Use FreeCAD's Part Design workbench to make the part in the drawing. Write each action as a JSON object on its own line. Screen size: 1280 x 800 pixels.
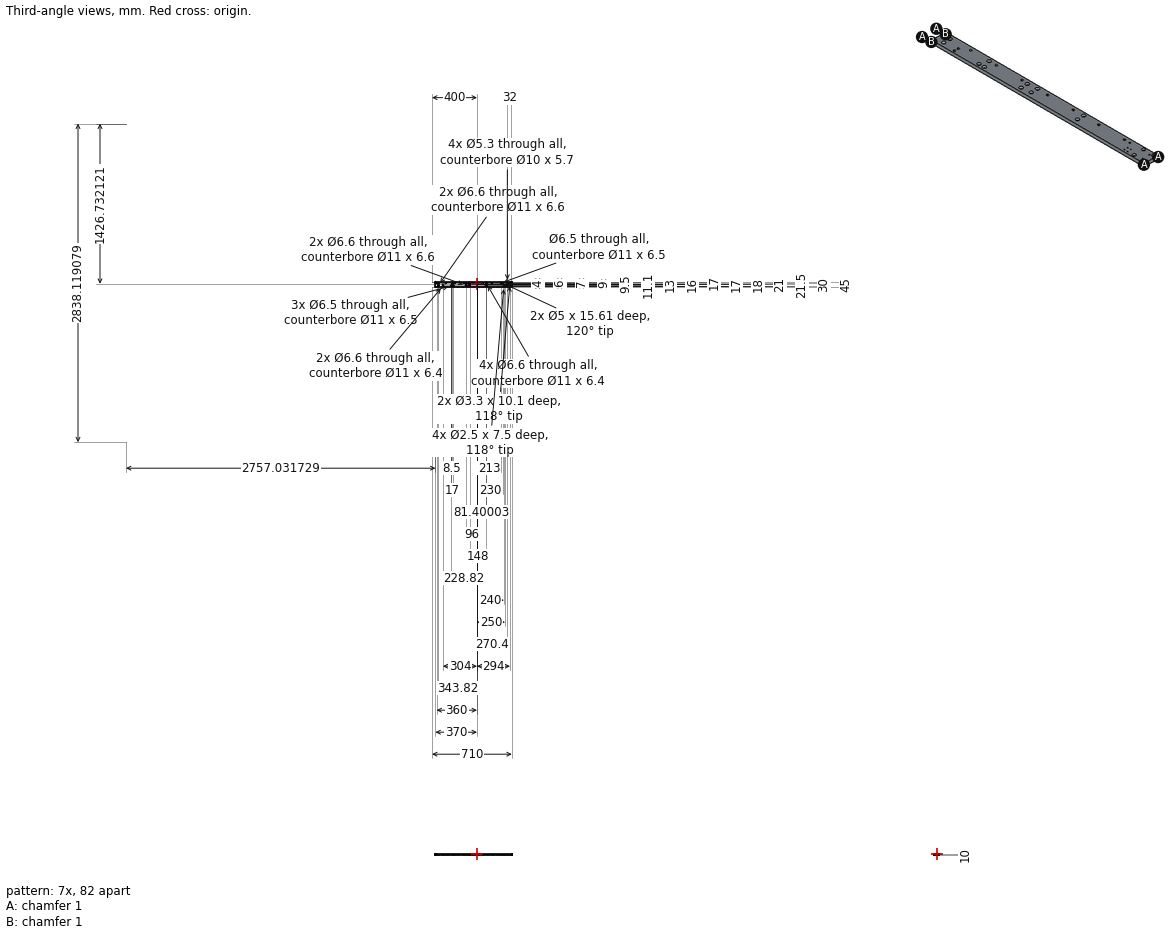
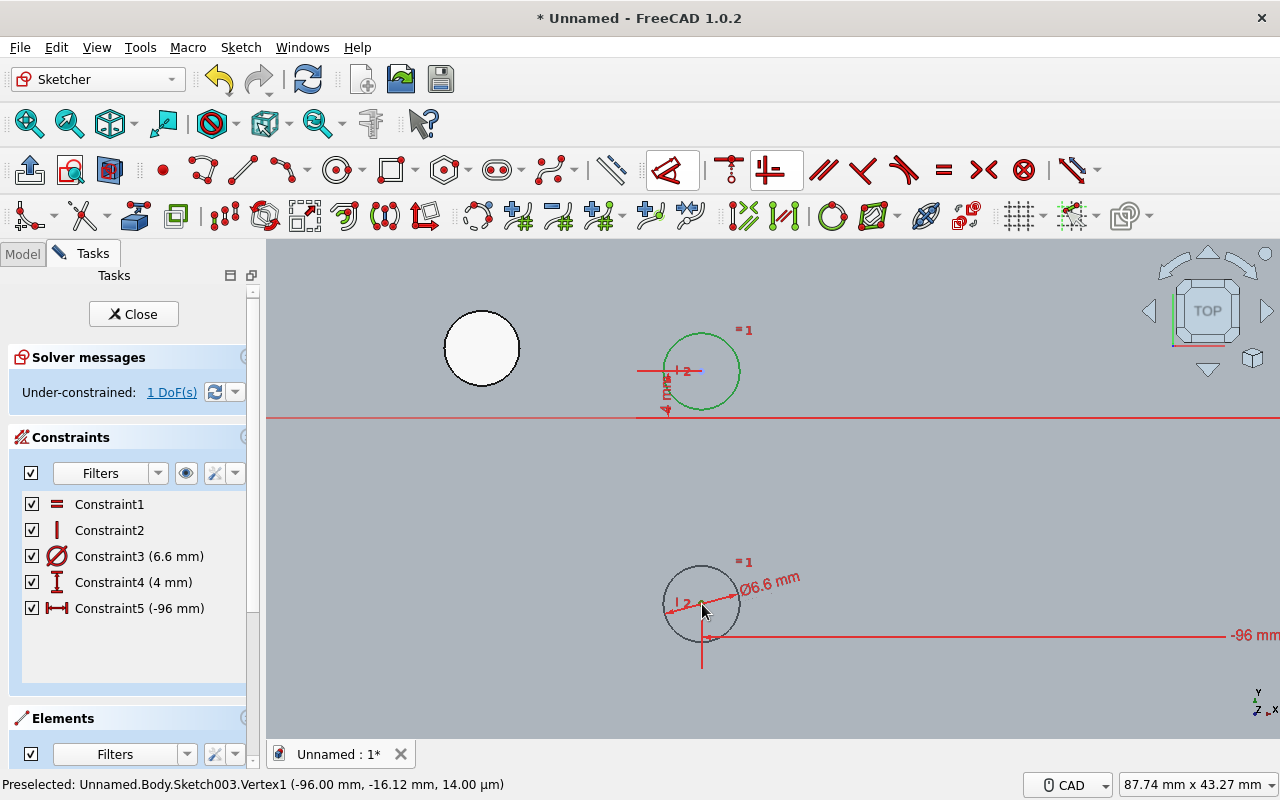
{"action": "left_click", "coordinate": [694, 170]}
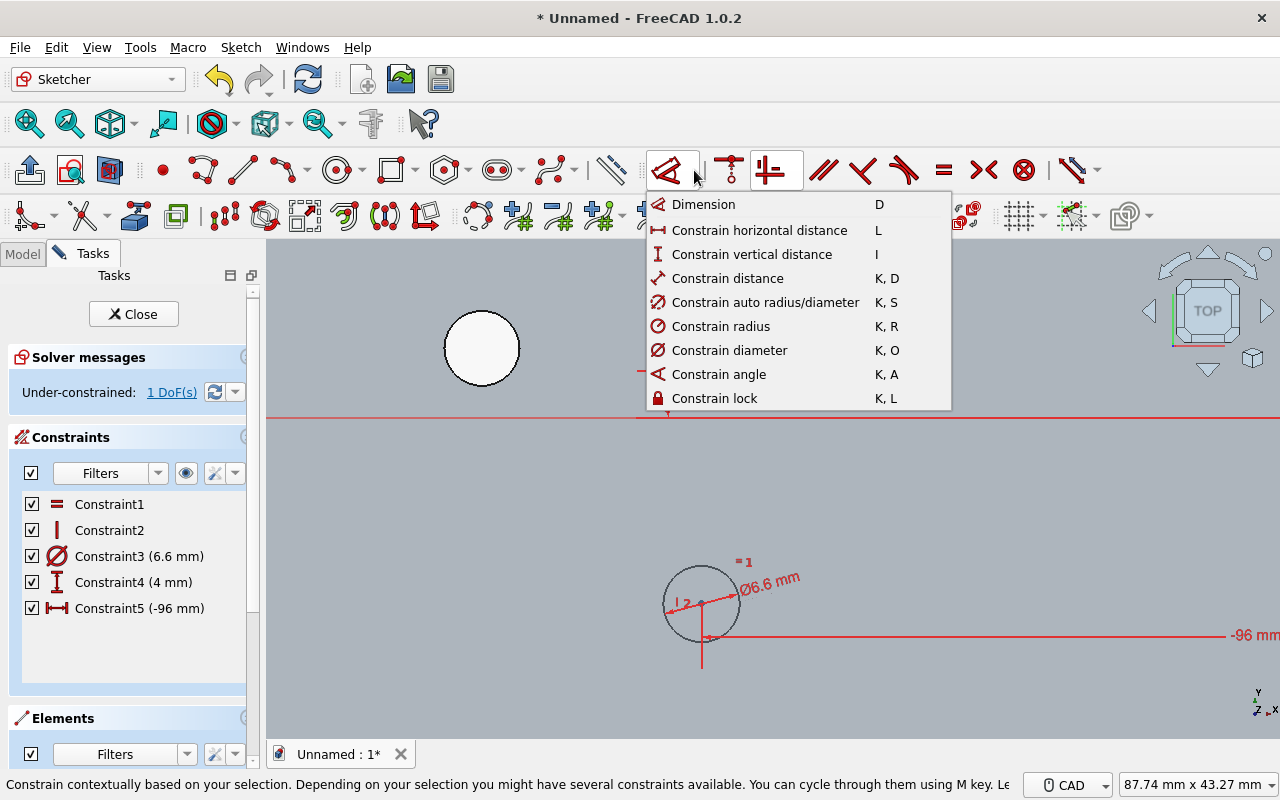
{"action": "left_click", "coordinate": [799, 254]}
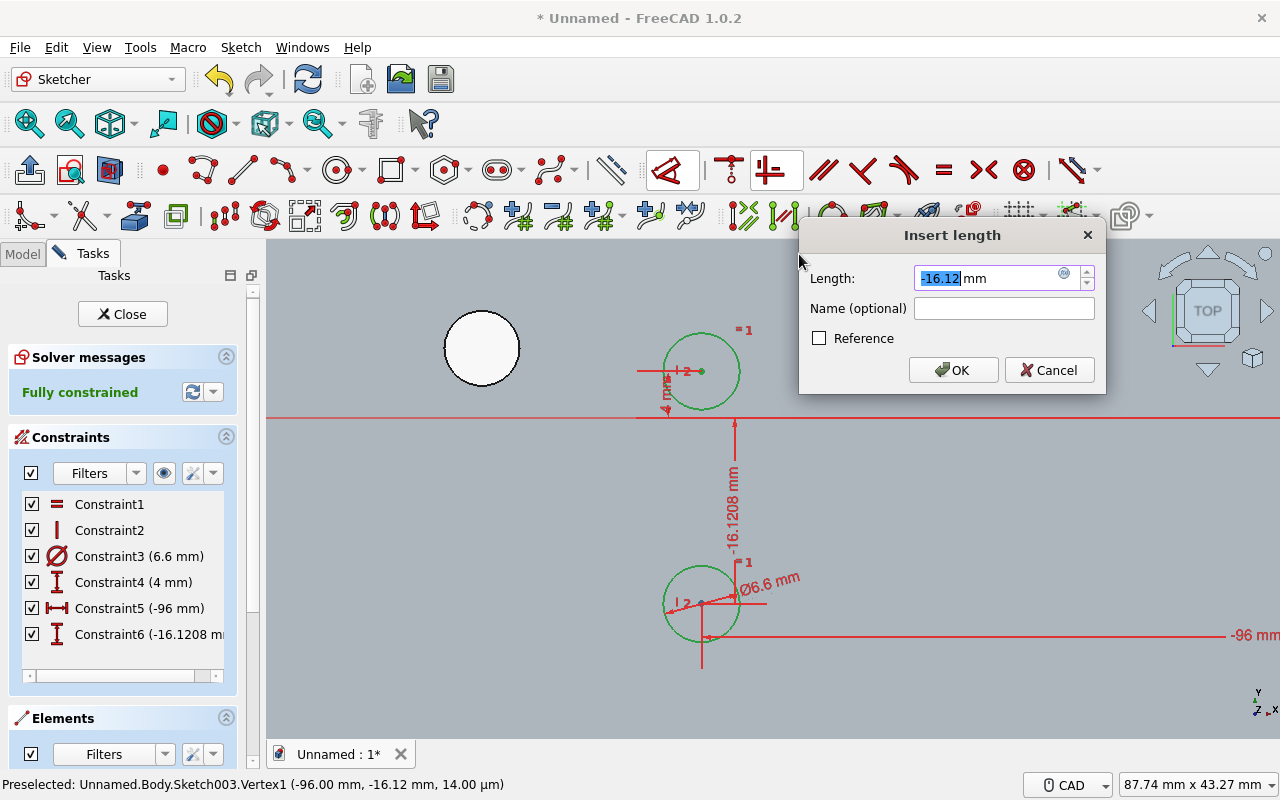
{"action": "type", "text": "-16"}
{"action": "key", "text": "Return"}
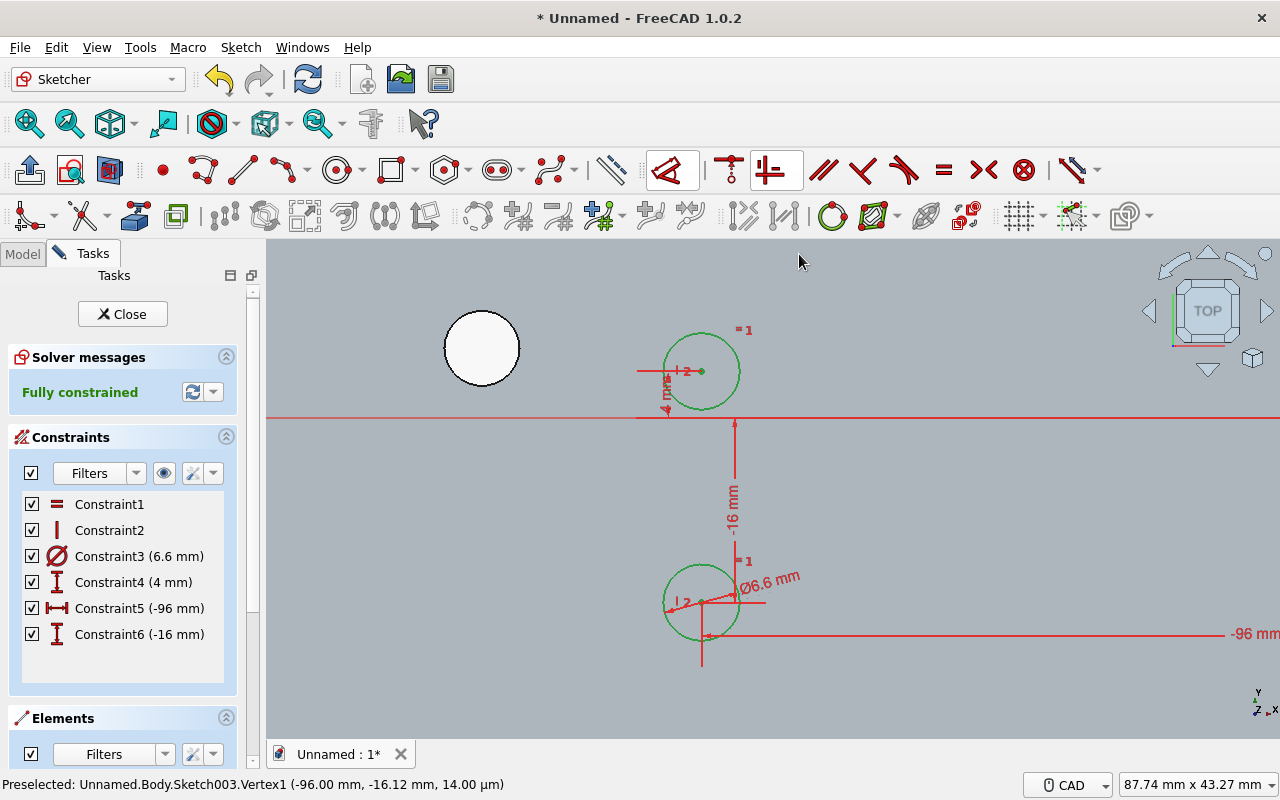
{"action": "left_click", "coordinate": [123, 314]}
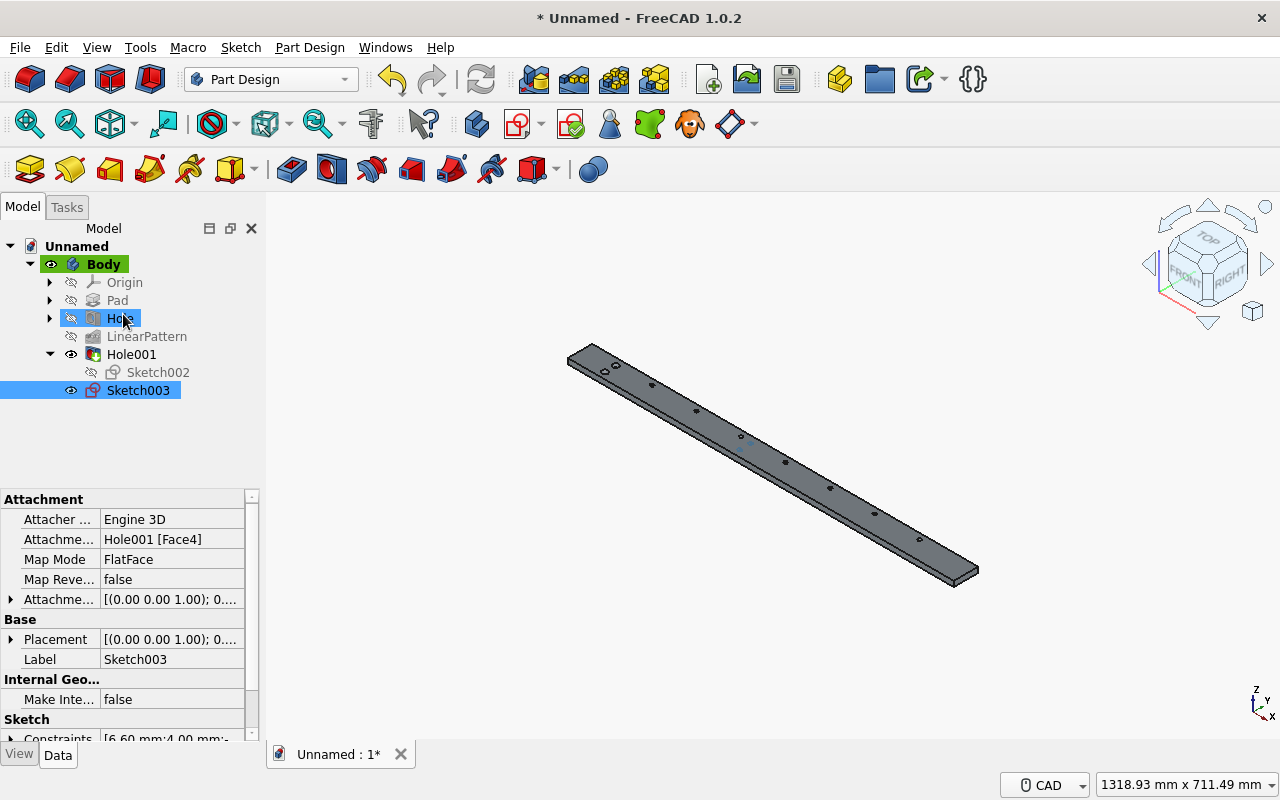
{"action": "left_click", "coordinate": [332, 170]}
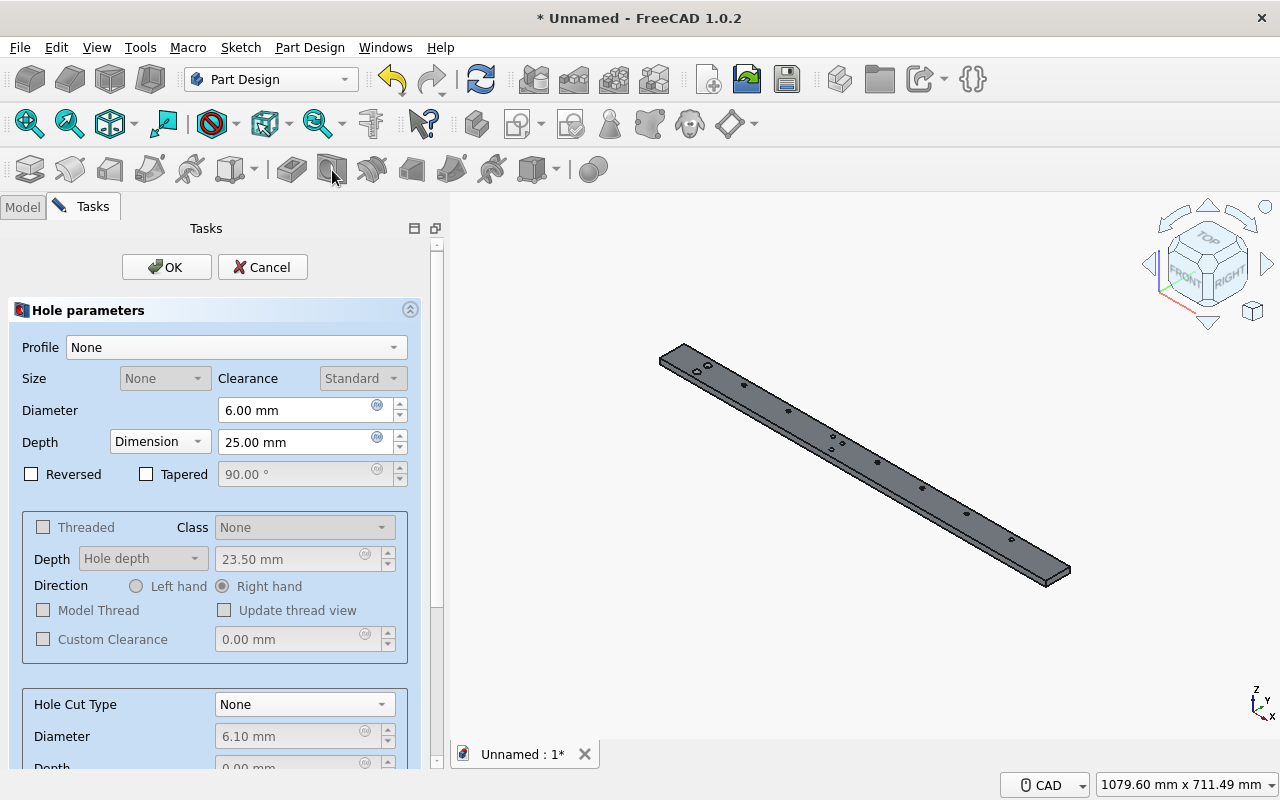
{"action": "triple_click", "coordinate": [305, 410]}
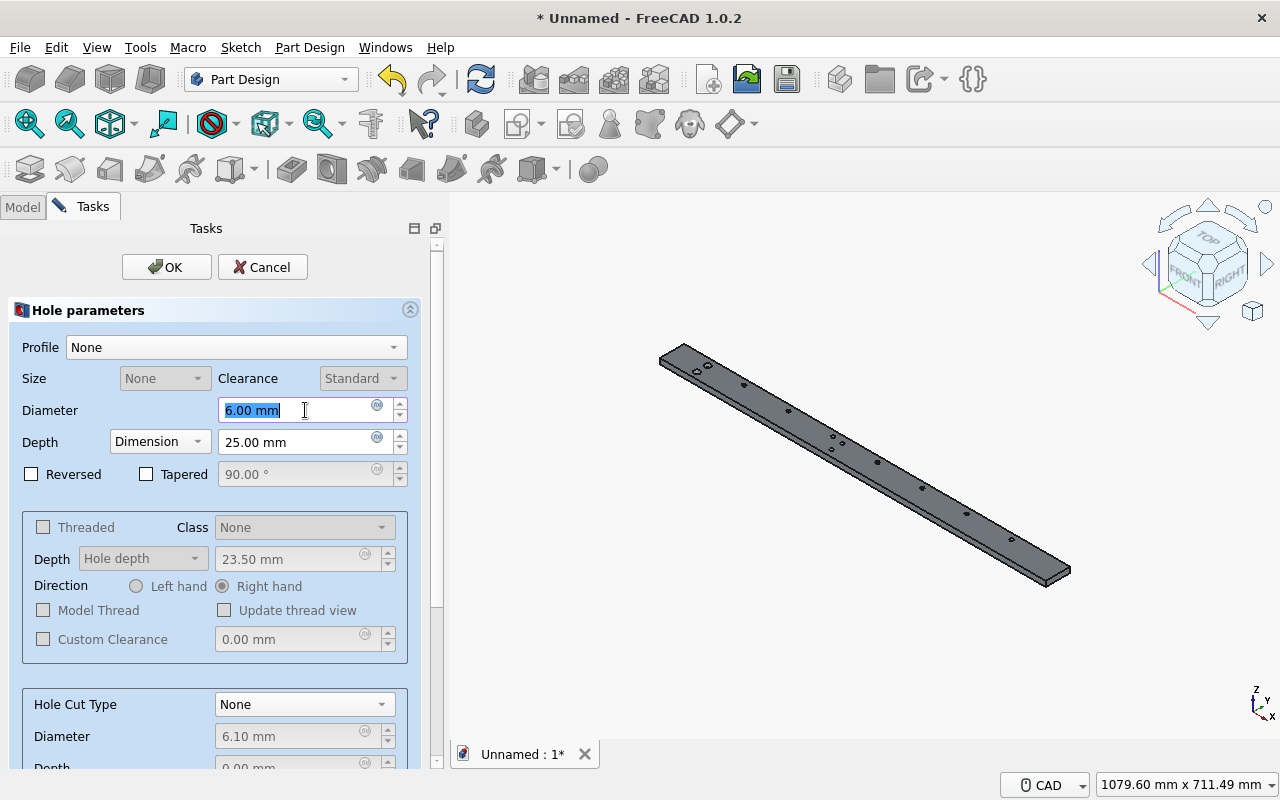
{"action": "type", "text": "6.6"}
{"action": "key", "text": "Tab"}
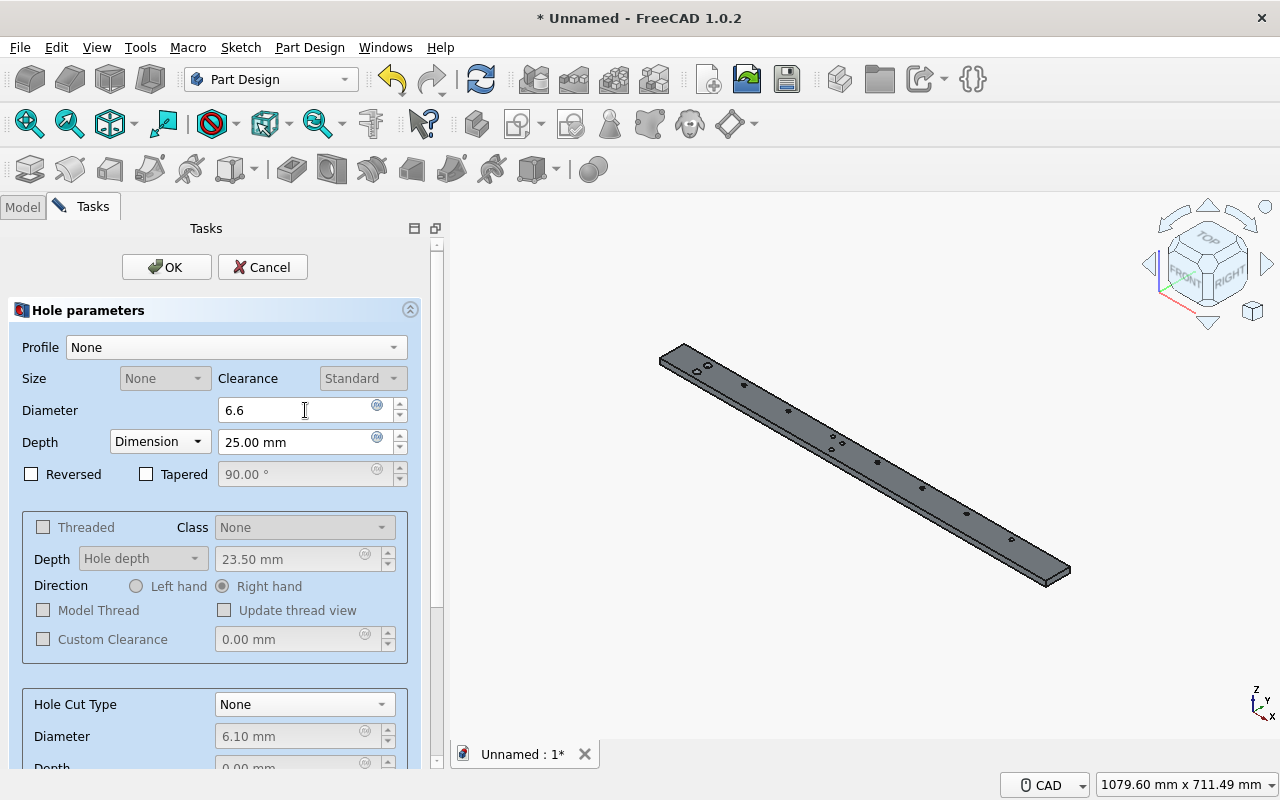
{"action": "left_click", "coordinate": [161, 442]}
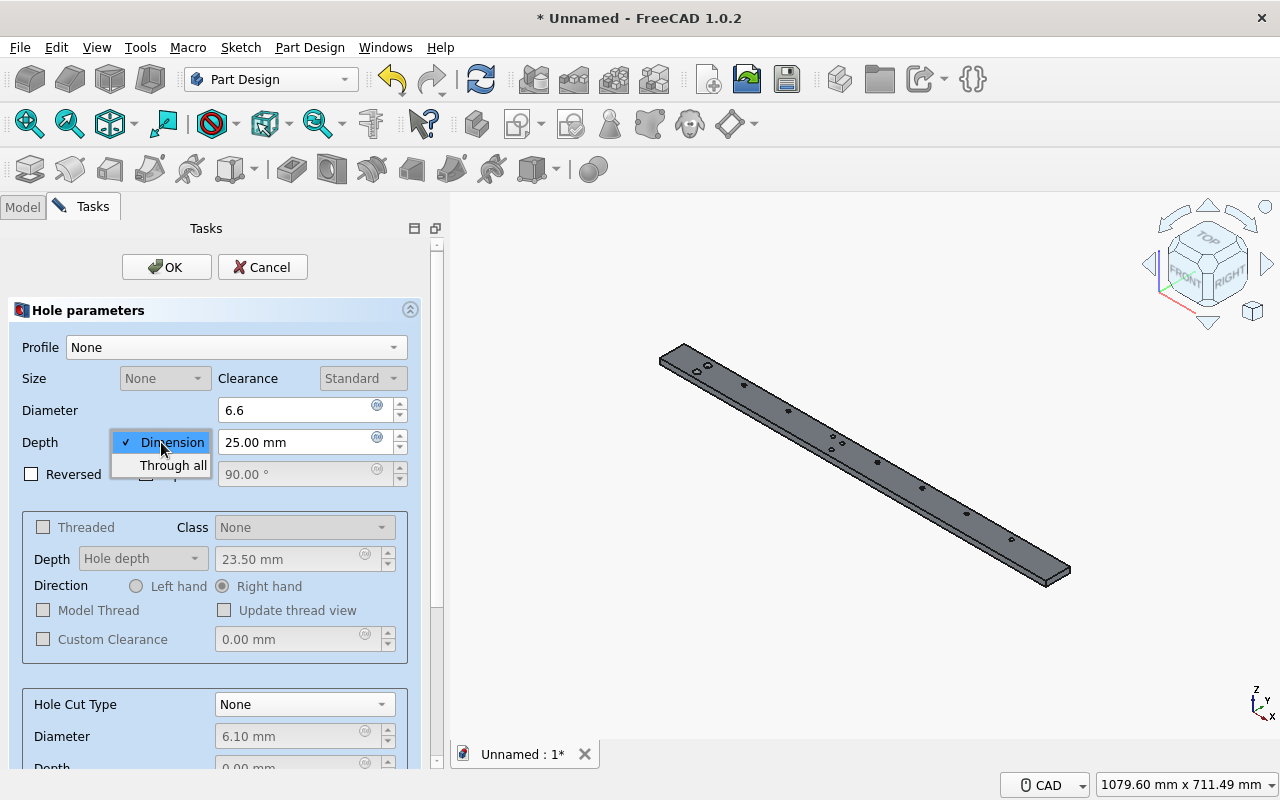
{"action": "left_click", "coordinate": [160, 466]}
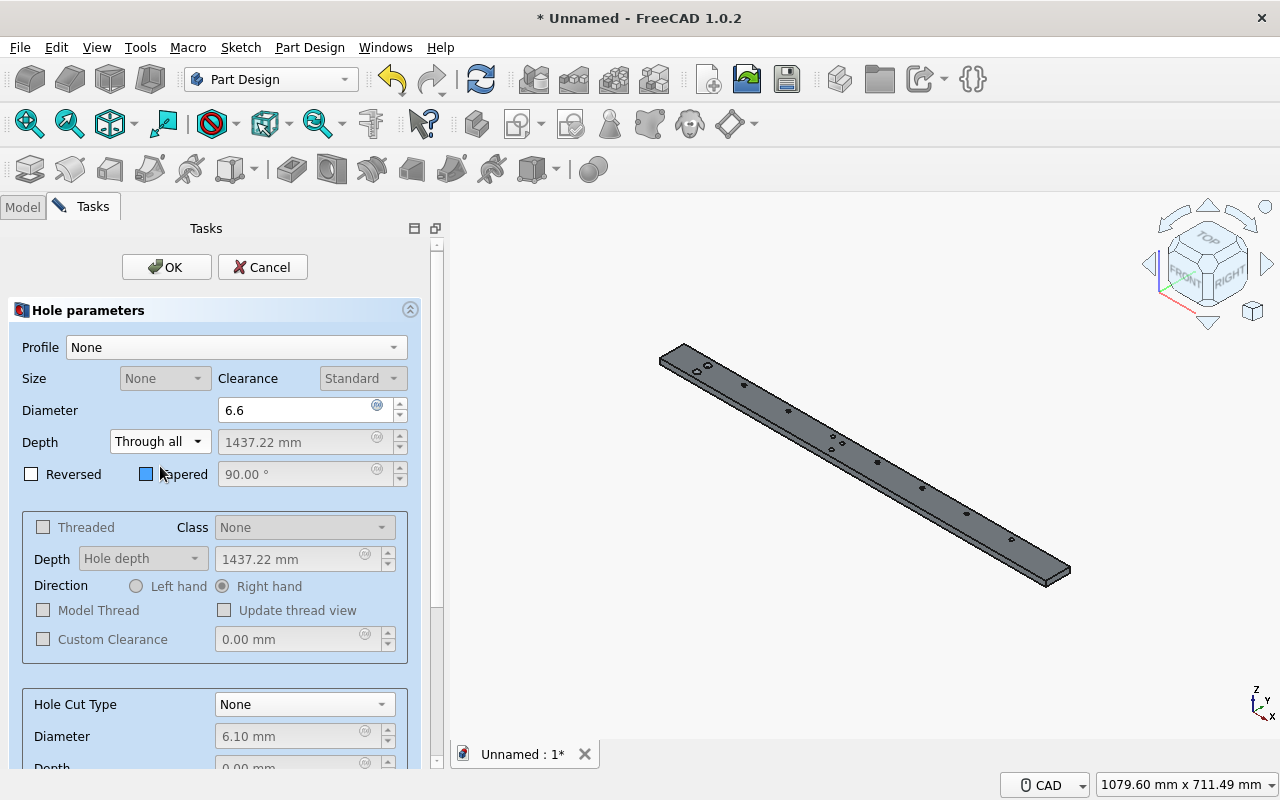
{"action": "left_click", "coordinate": [306, 704]}